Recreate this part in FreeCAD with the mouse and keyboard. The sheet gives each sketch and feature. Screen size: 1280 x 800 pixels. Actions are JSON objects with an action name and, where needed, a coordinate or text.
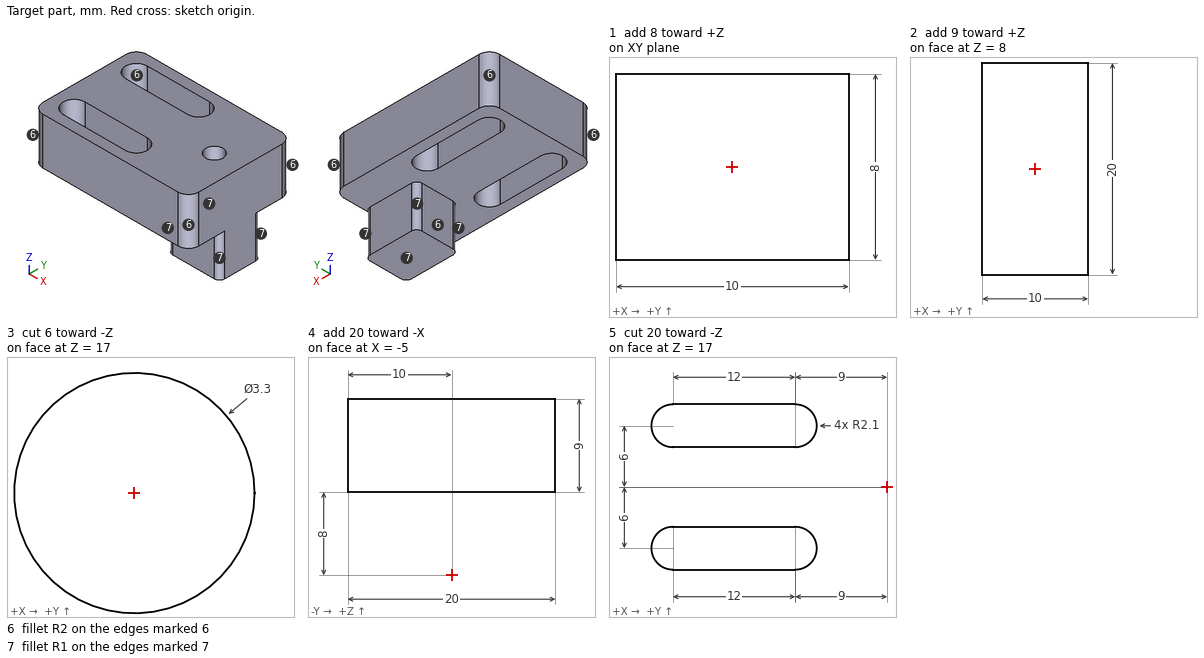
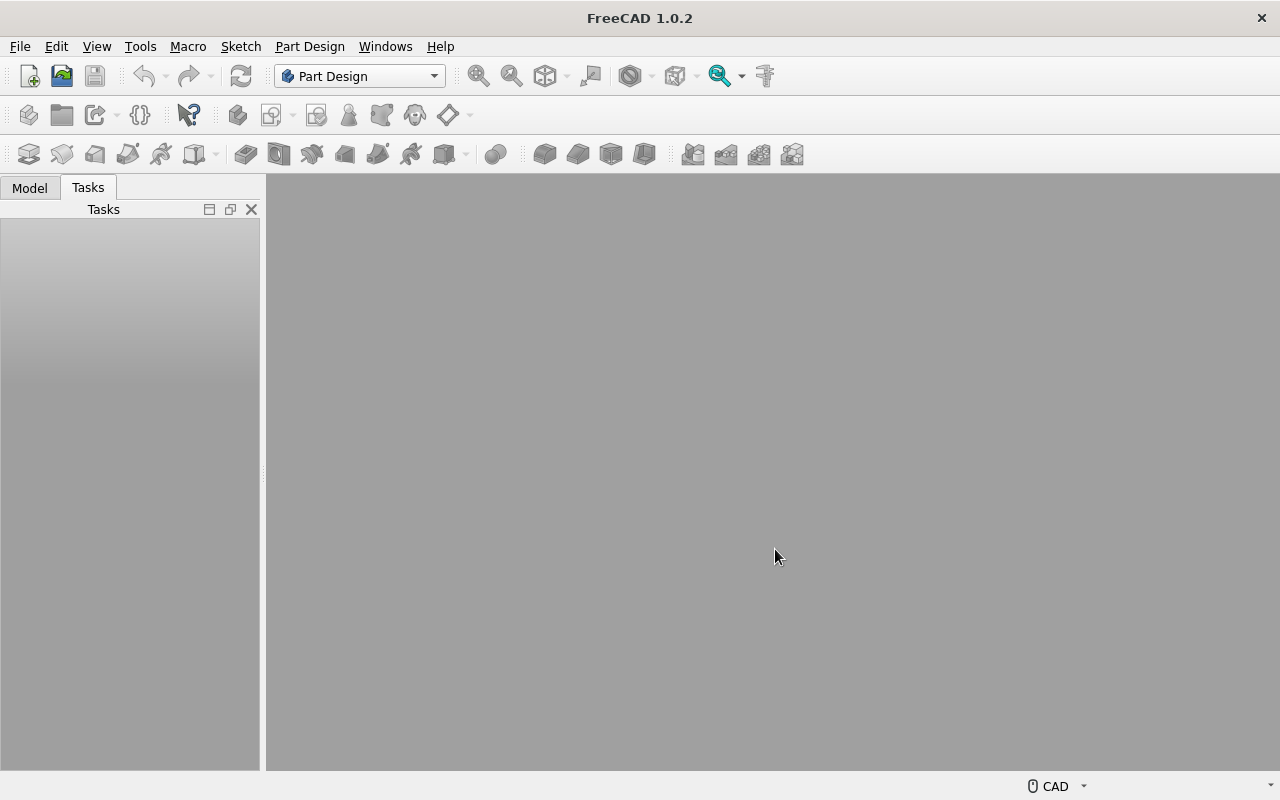
{"action": "left_click", "coordinate": [29, 76]}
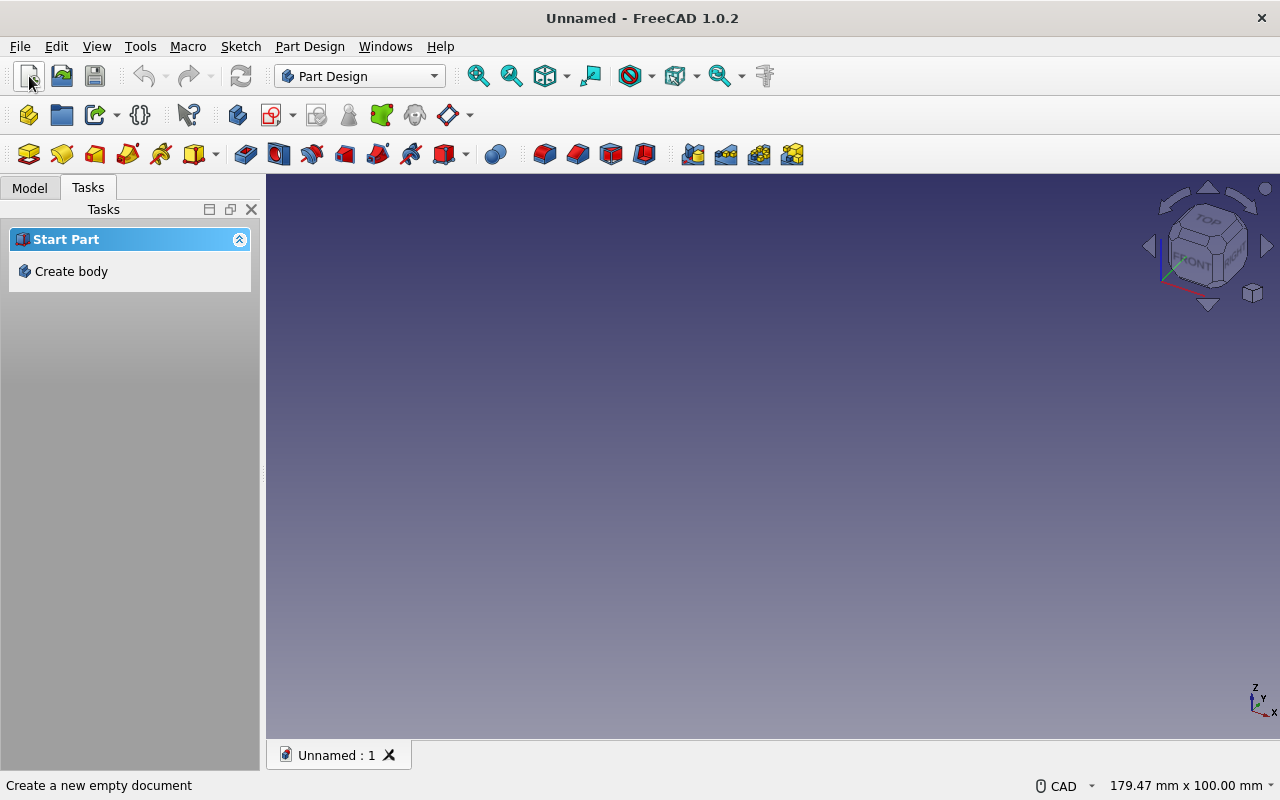
{"action": "left_click", "coordinate": [270, 116]}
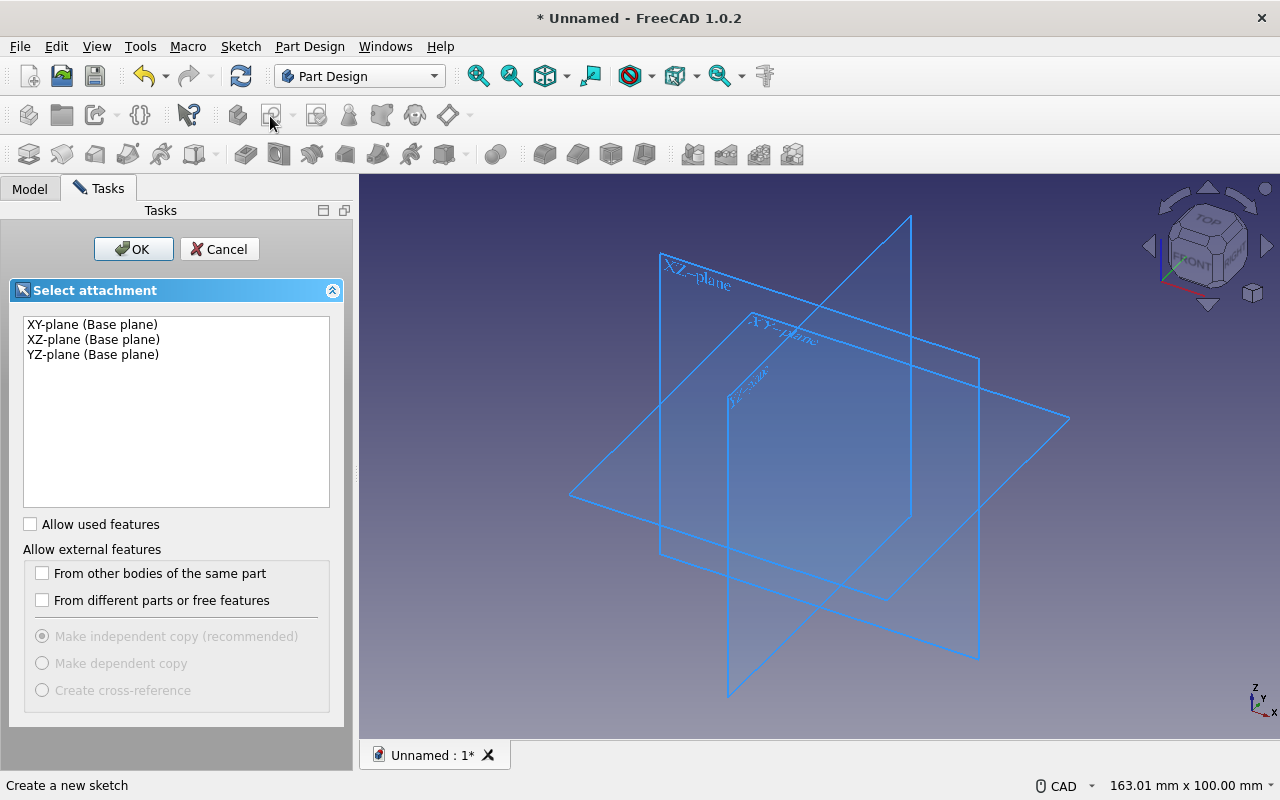
{"action": "left_click", "coordinate": [84, 324]}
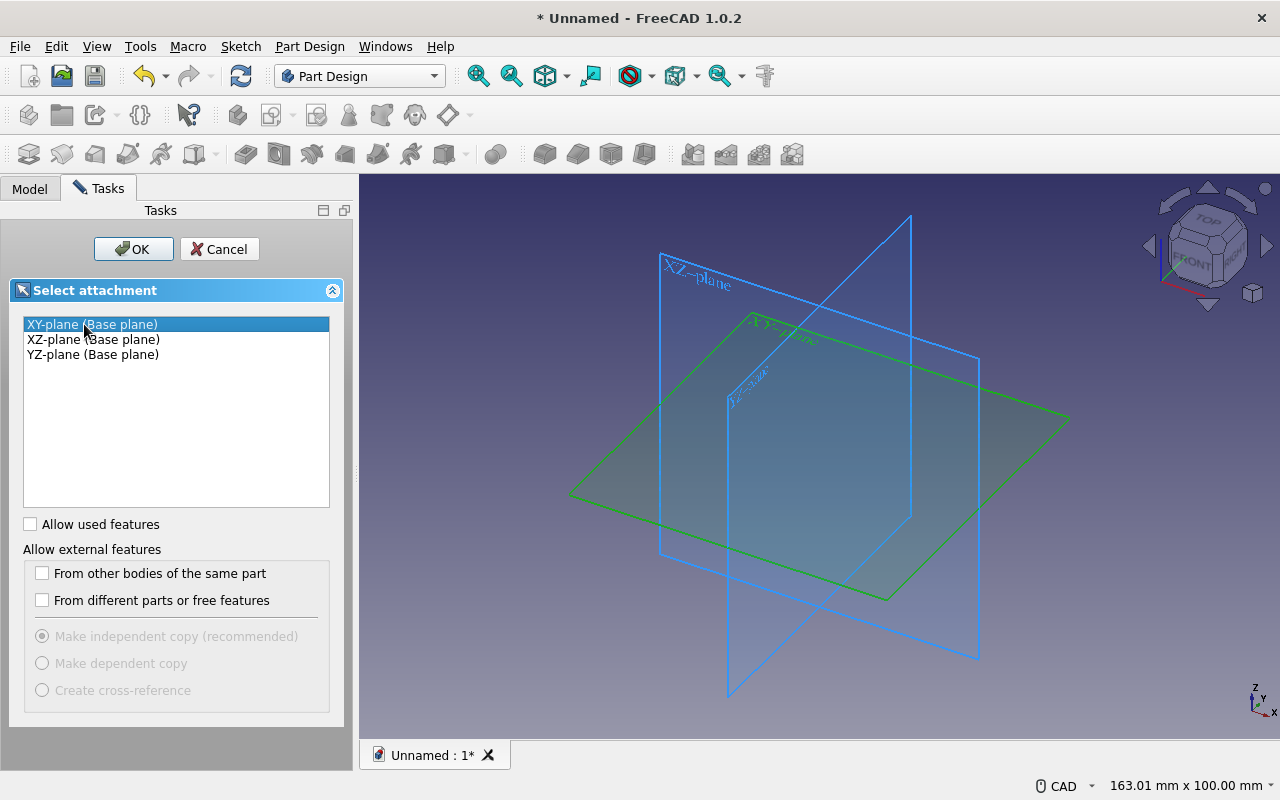
{"action": "left_click", "coordinate": [134, 249]}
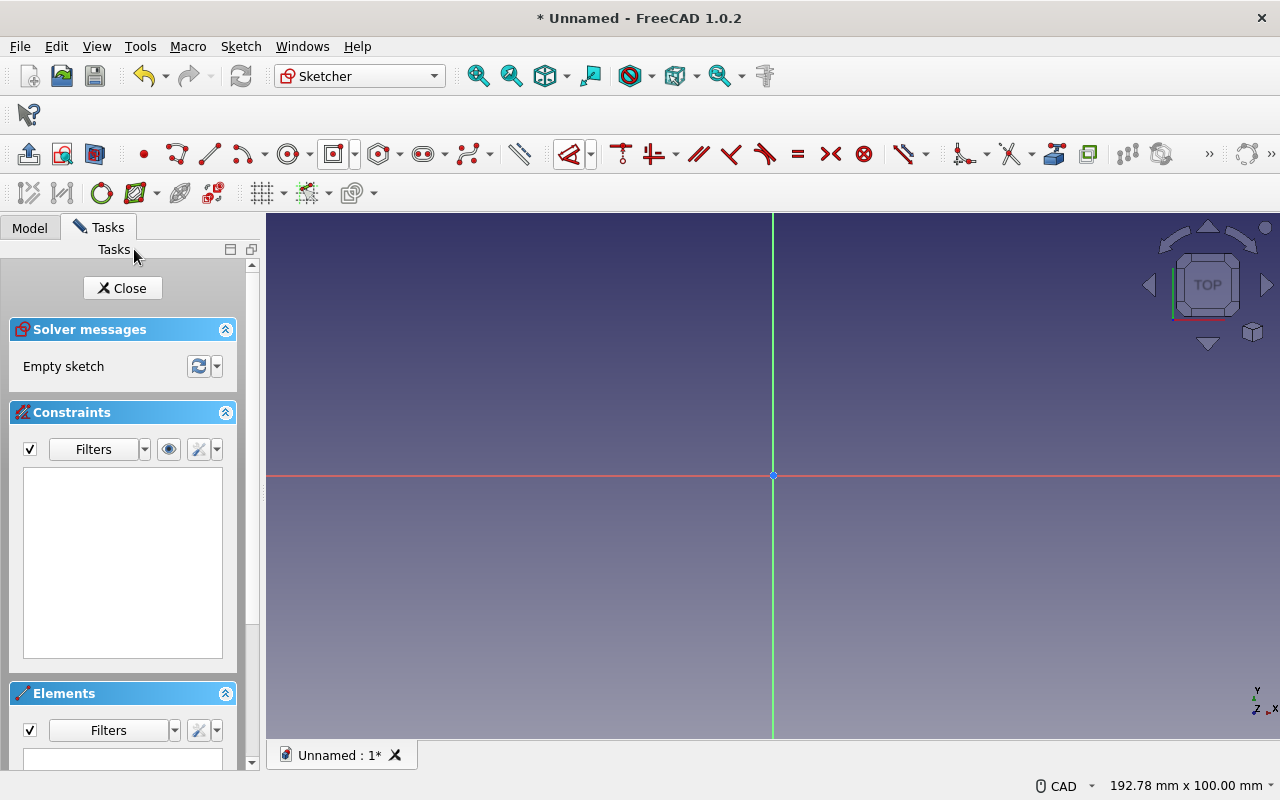
{"action": "scroll", "coordinate": [784, 476], "scroll_direction": "up", "scroll_amount": 10}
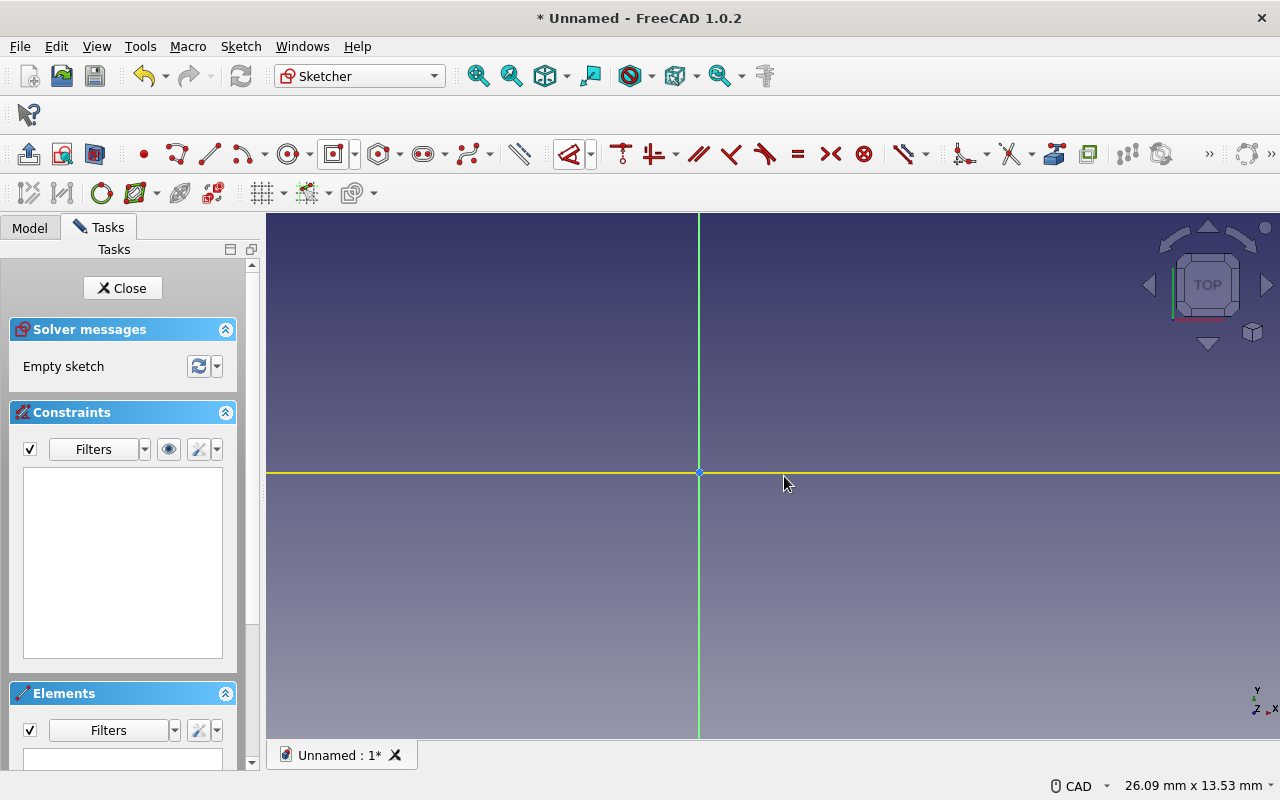
{"action": "left_click", "coordinate": [332, 154]}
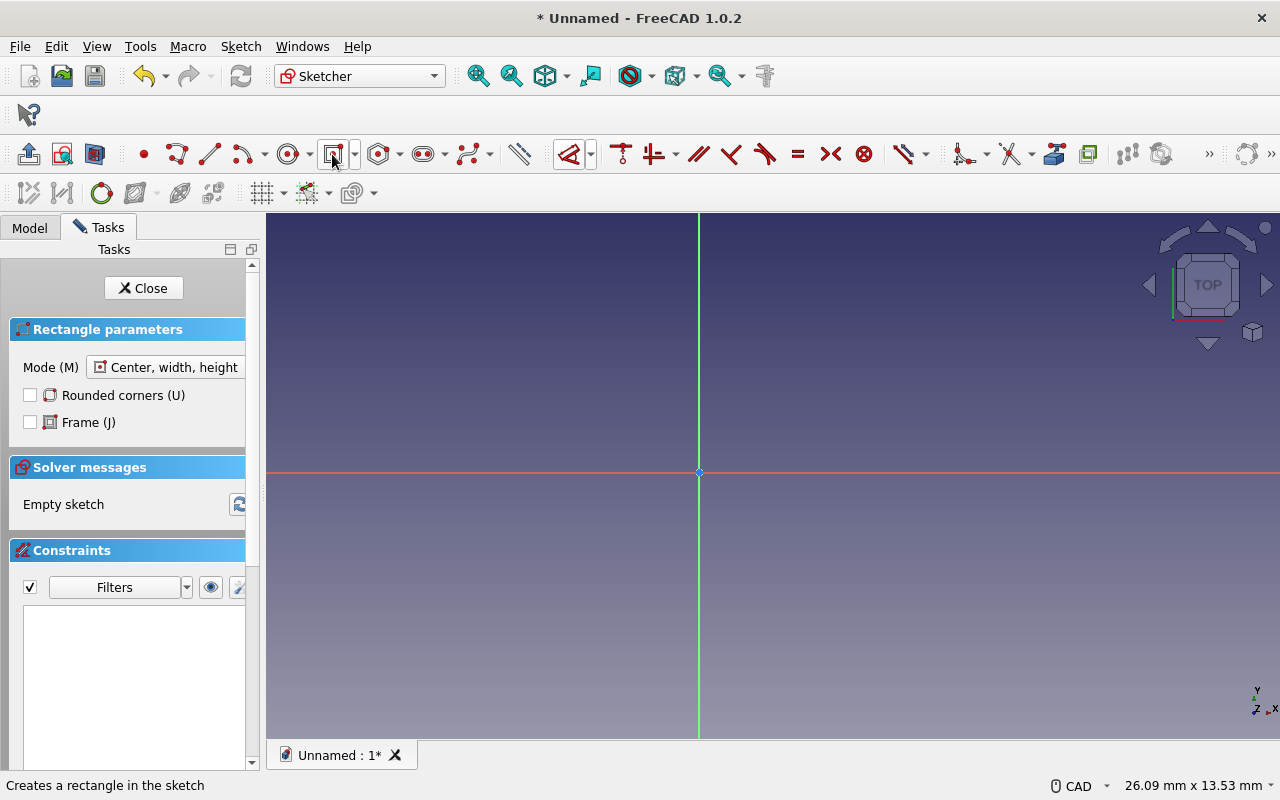
{"action": "left_click", "coordinate": [699, 473]}
{"action": "mouse_move", "coordinate": [894, 317]}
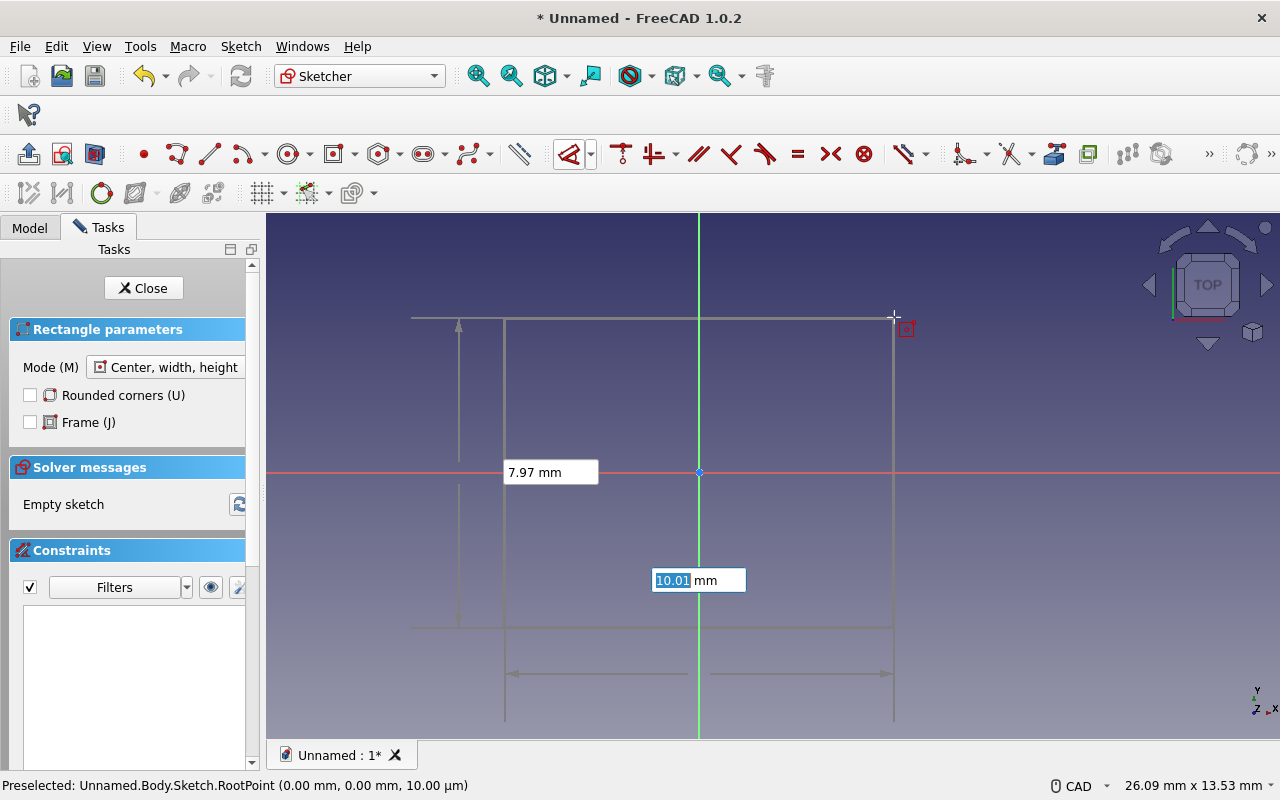
{"action": "type", "text": "10"}
{"action": "key", "text": "Tab"}
{"action": "type", "text": "8"}
{"action": "key", "text": "Return"}
{"action": "key", "text": "Escape"}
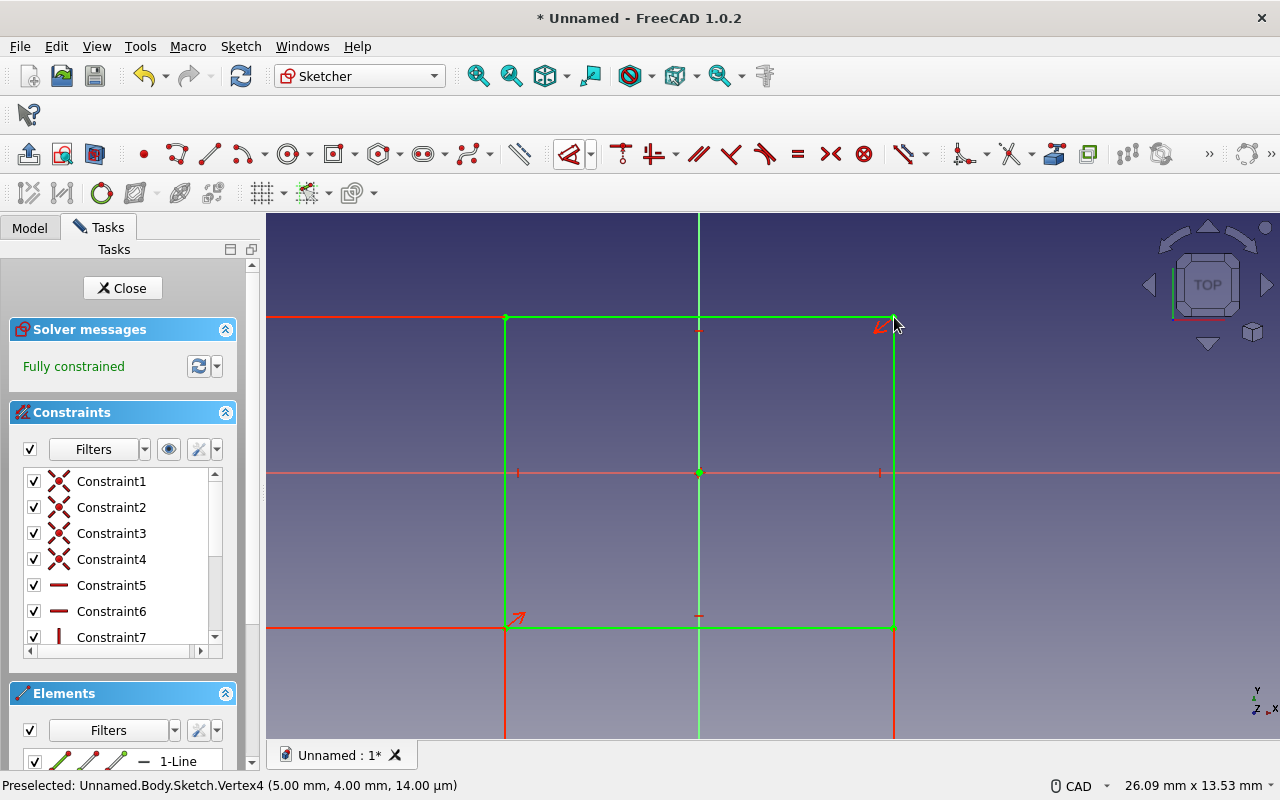
{"action": "left_click", "coordinate": [123, 288]}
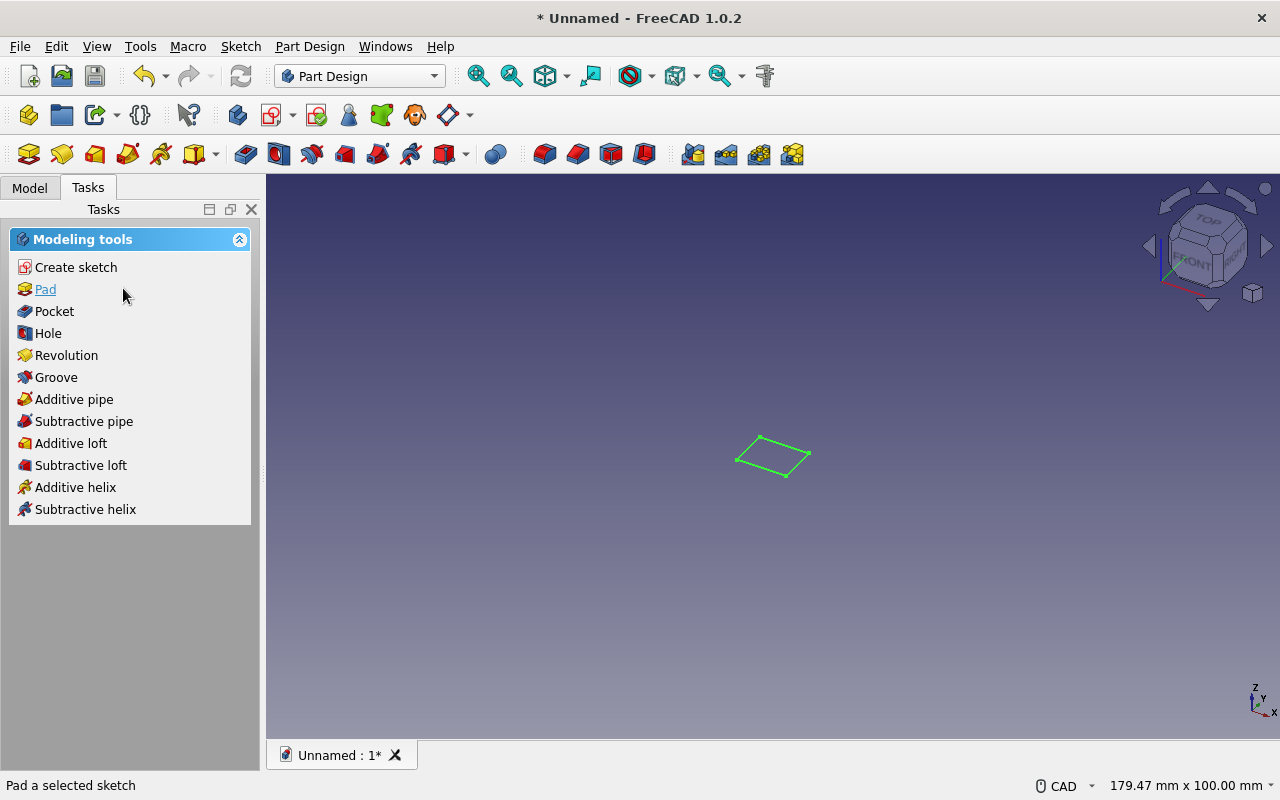
{"action": "left_click", "coordinate": [29, 154]}